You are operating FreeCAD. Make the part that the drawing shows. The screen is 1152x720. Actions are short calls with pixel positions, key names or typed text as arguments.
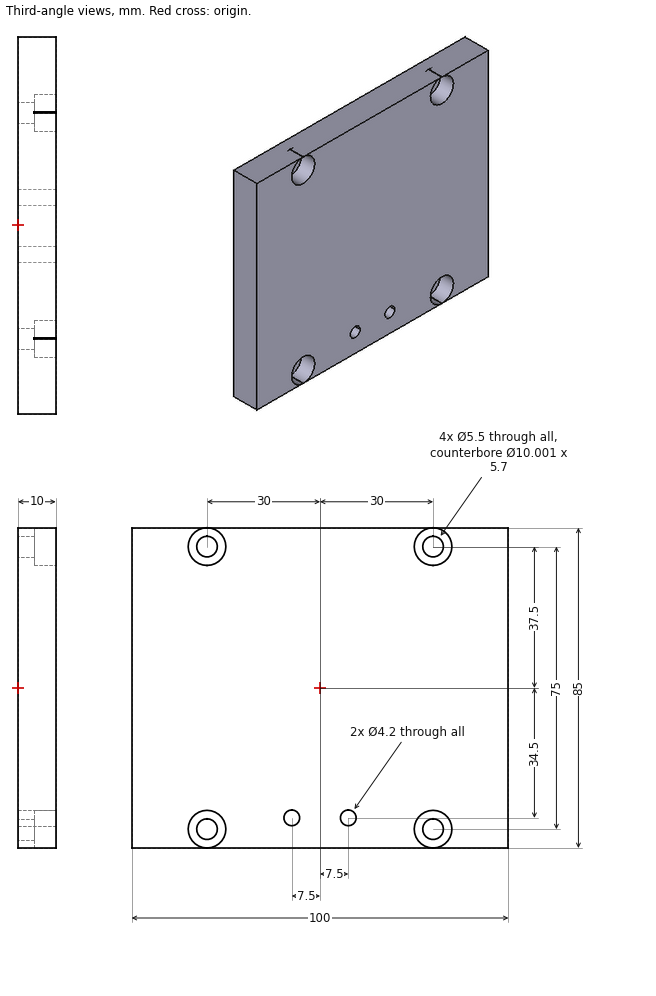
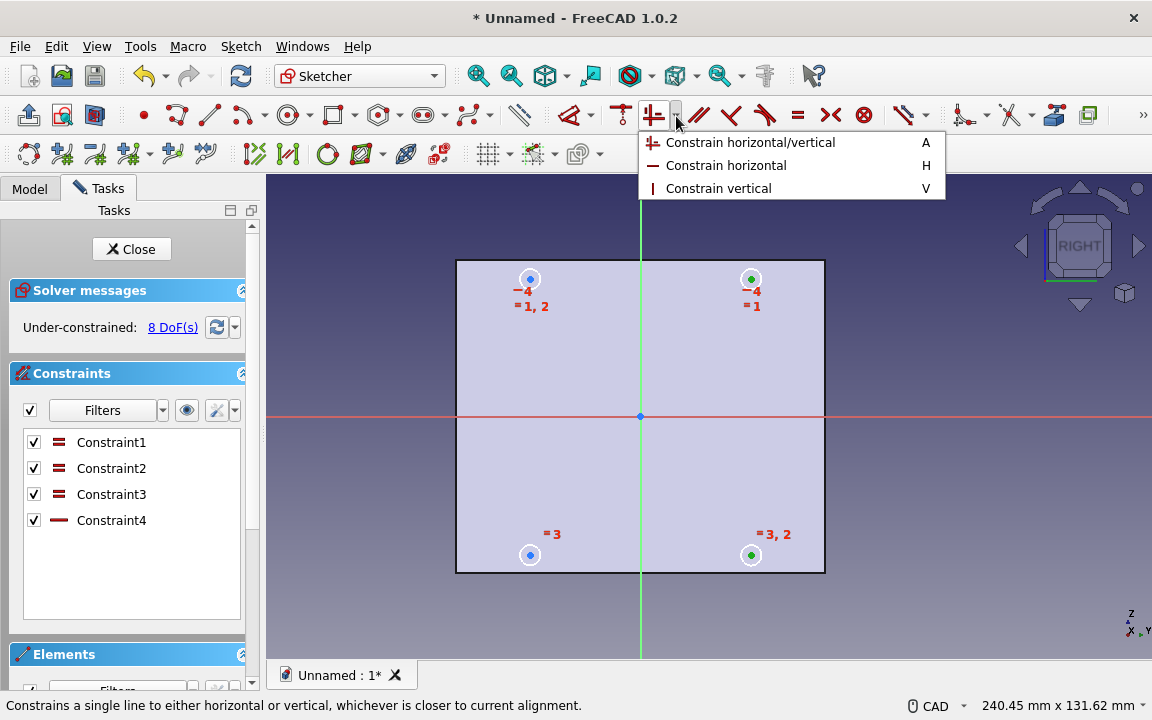
click(792, 188)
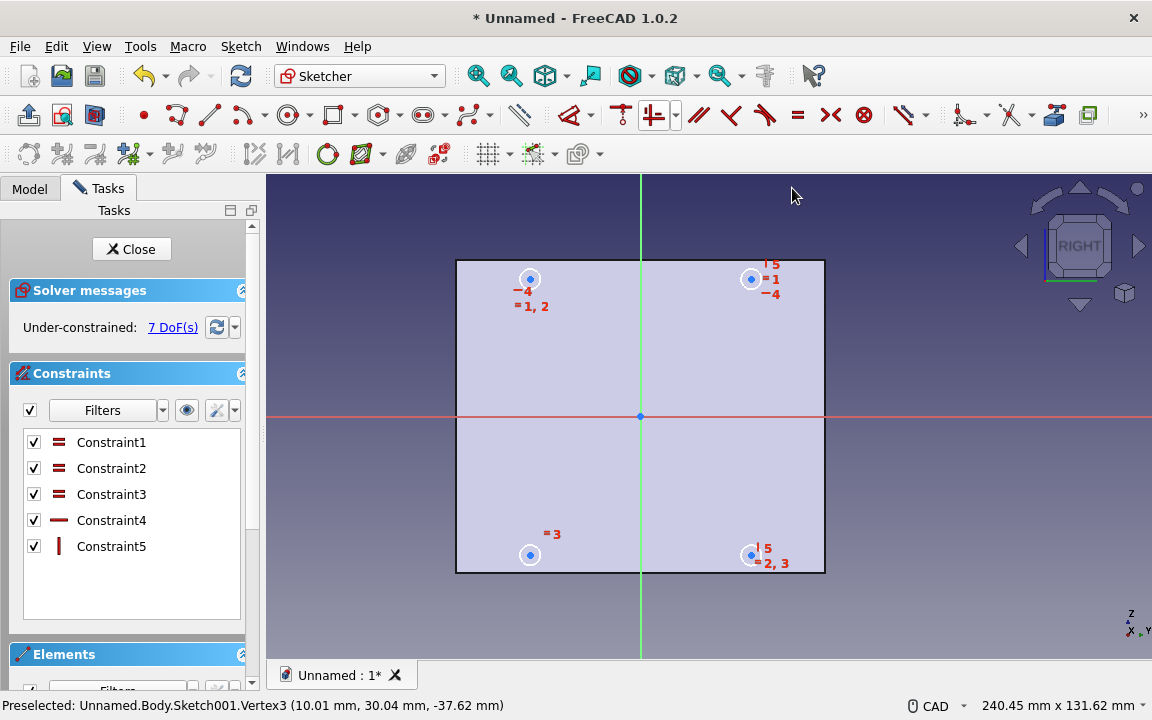
click(530, 279)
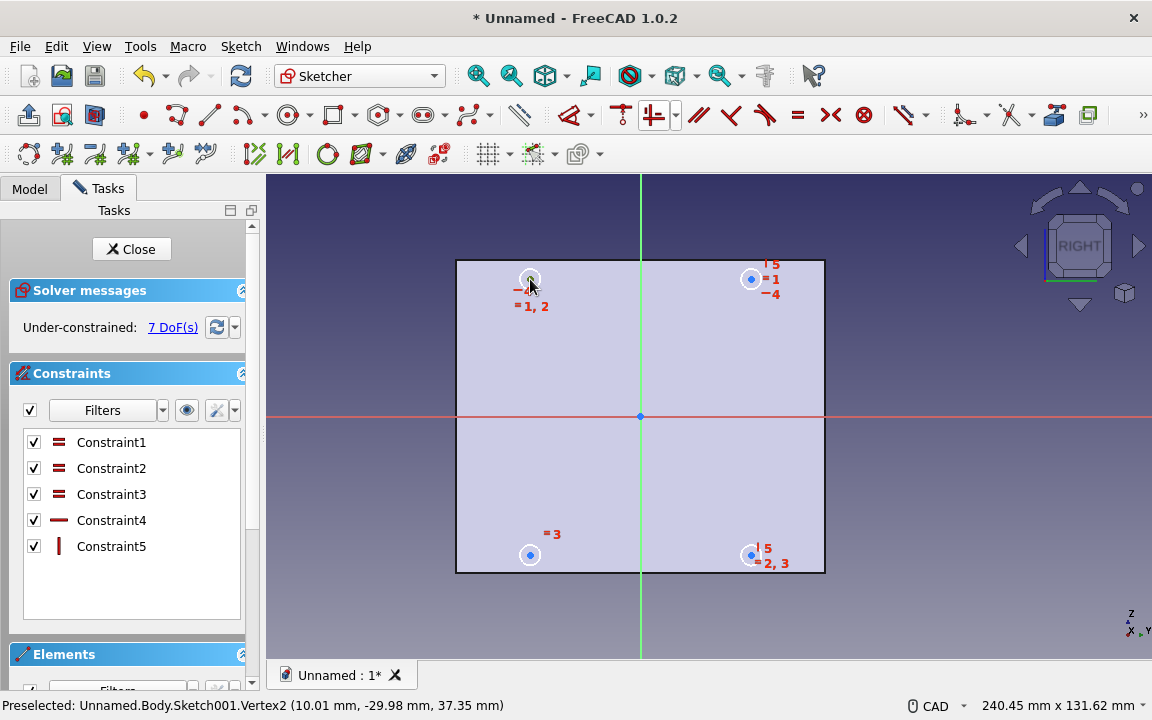
click(530, 555)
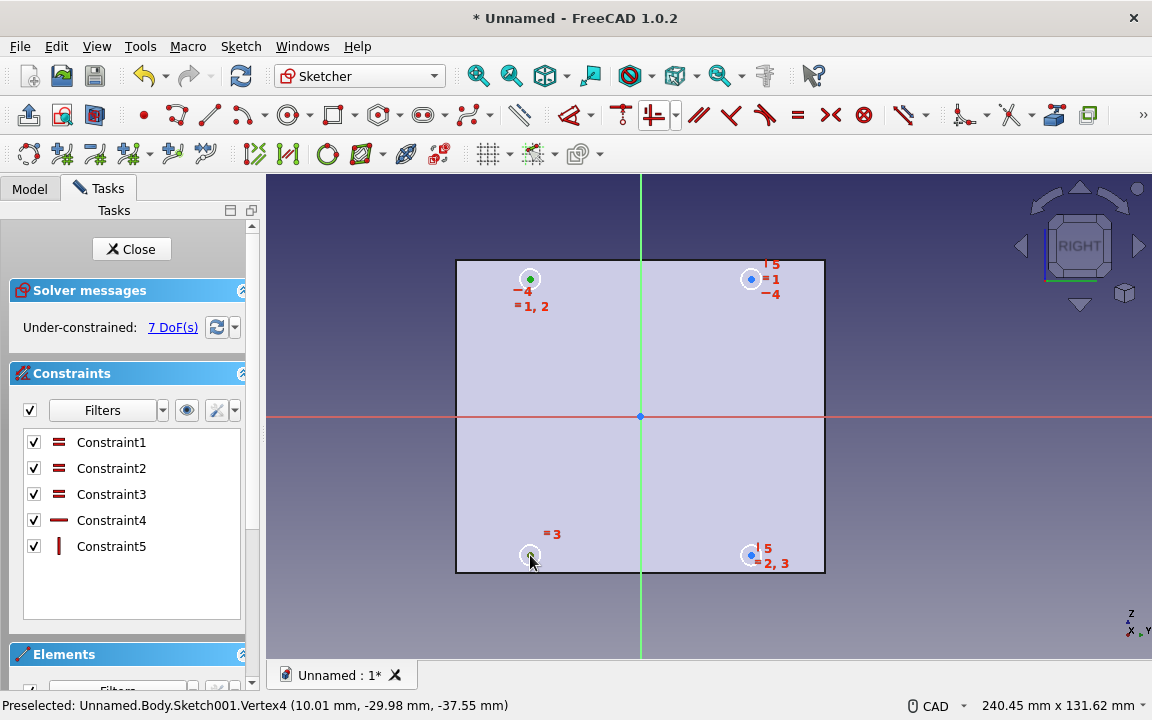
click(676, 116)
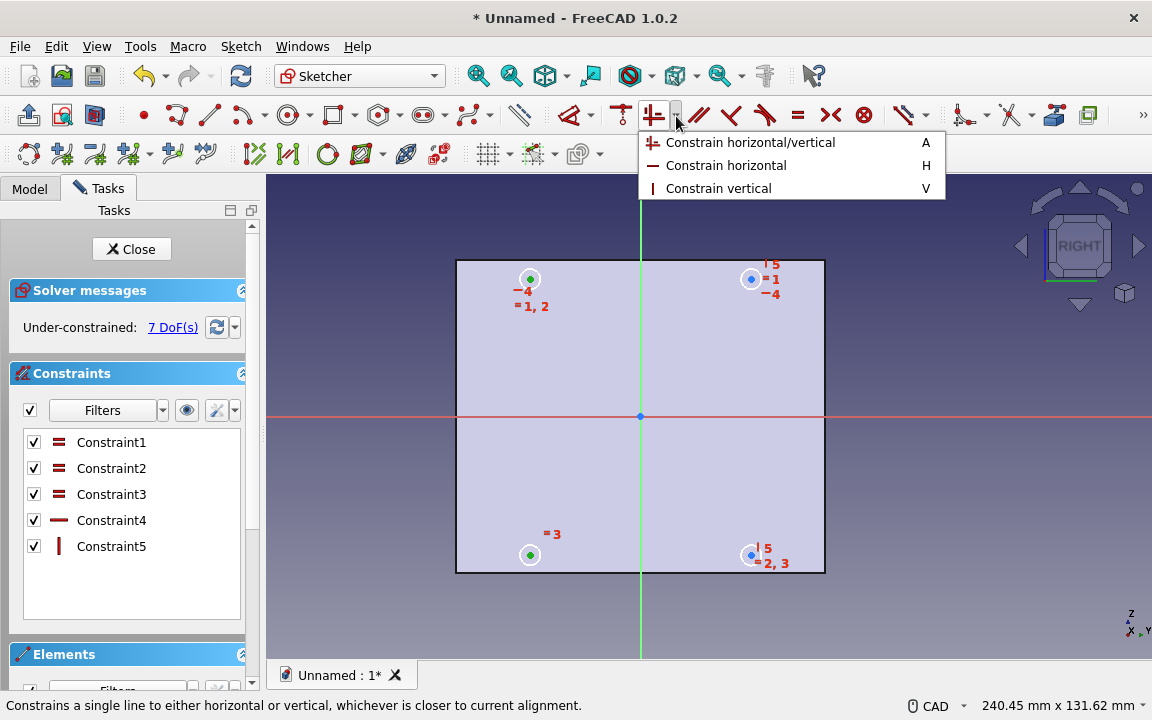
click(792, 188)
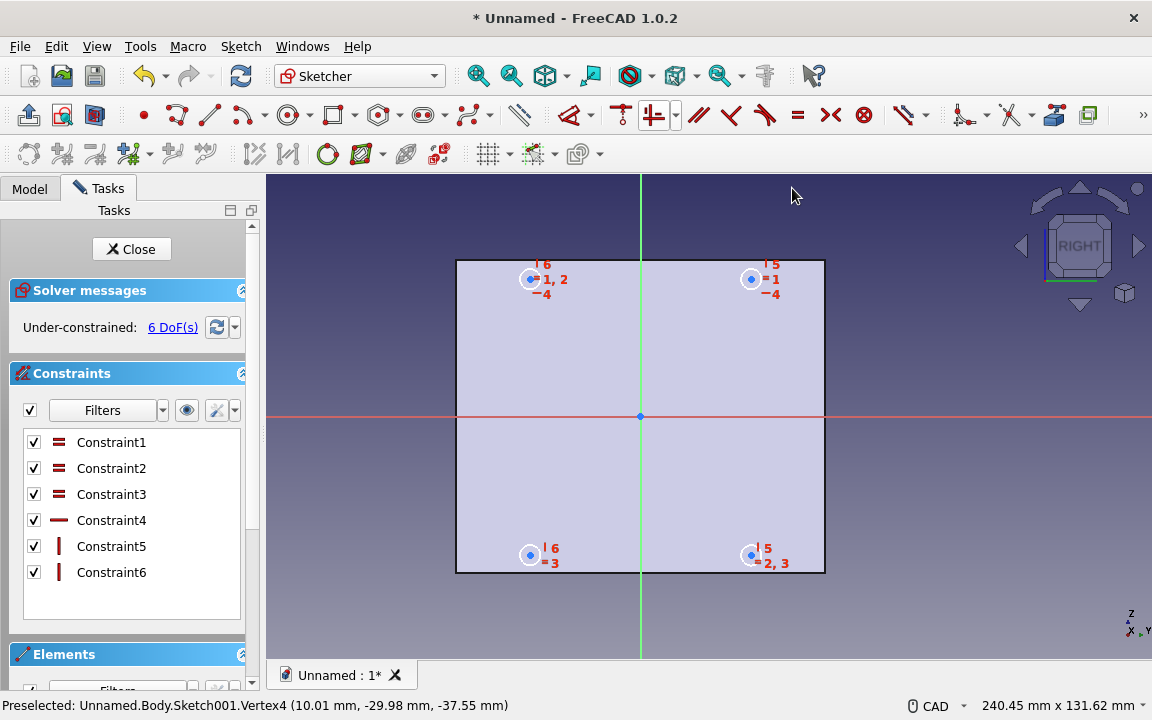
click(751, 555)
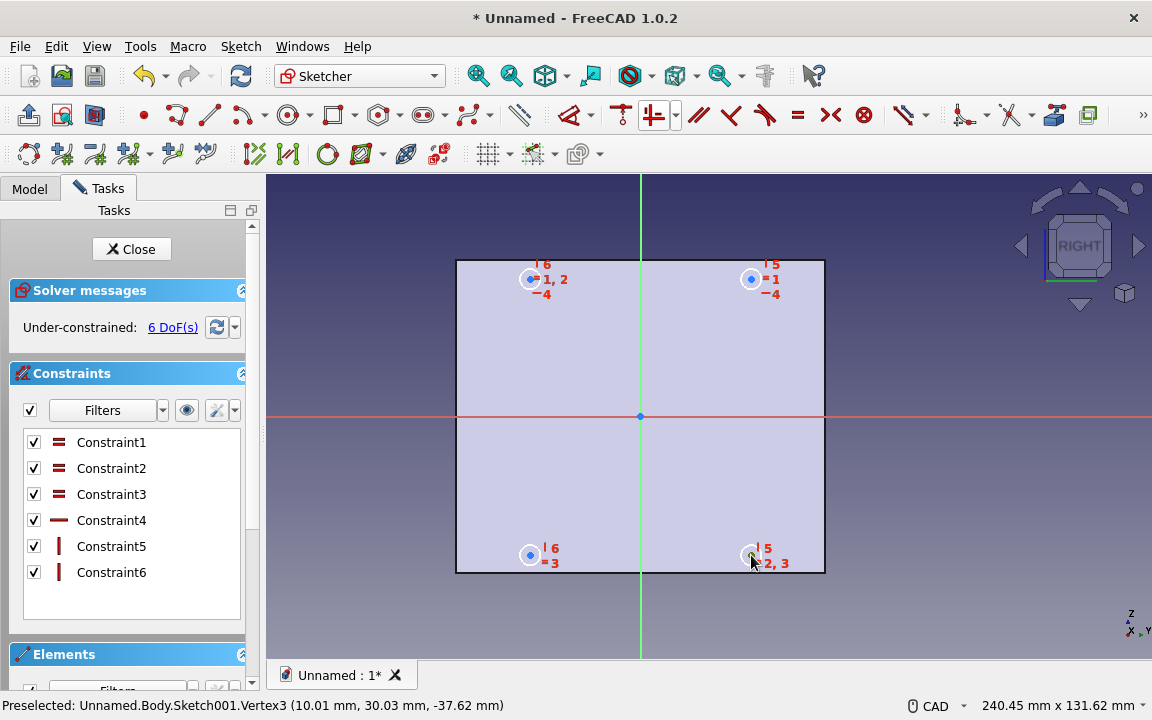
click(530, 555)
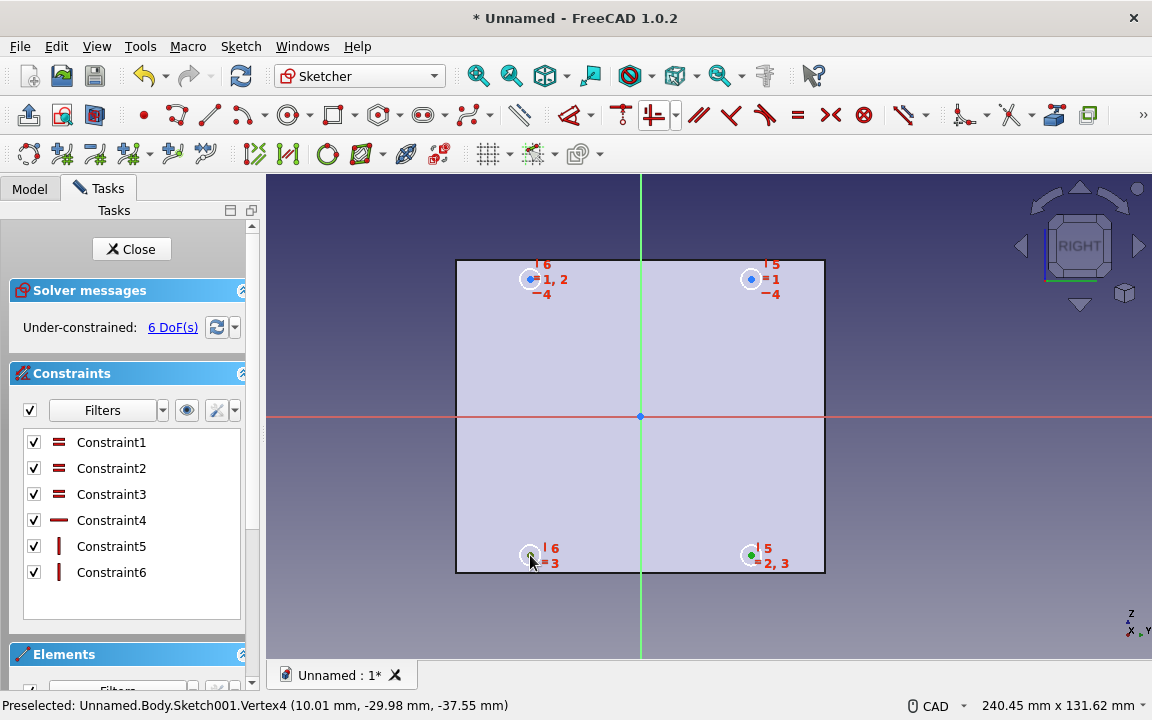
click(676, 116)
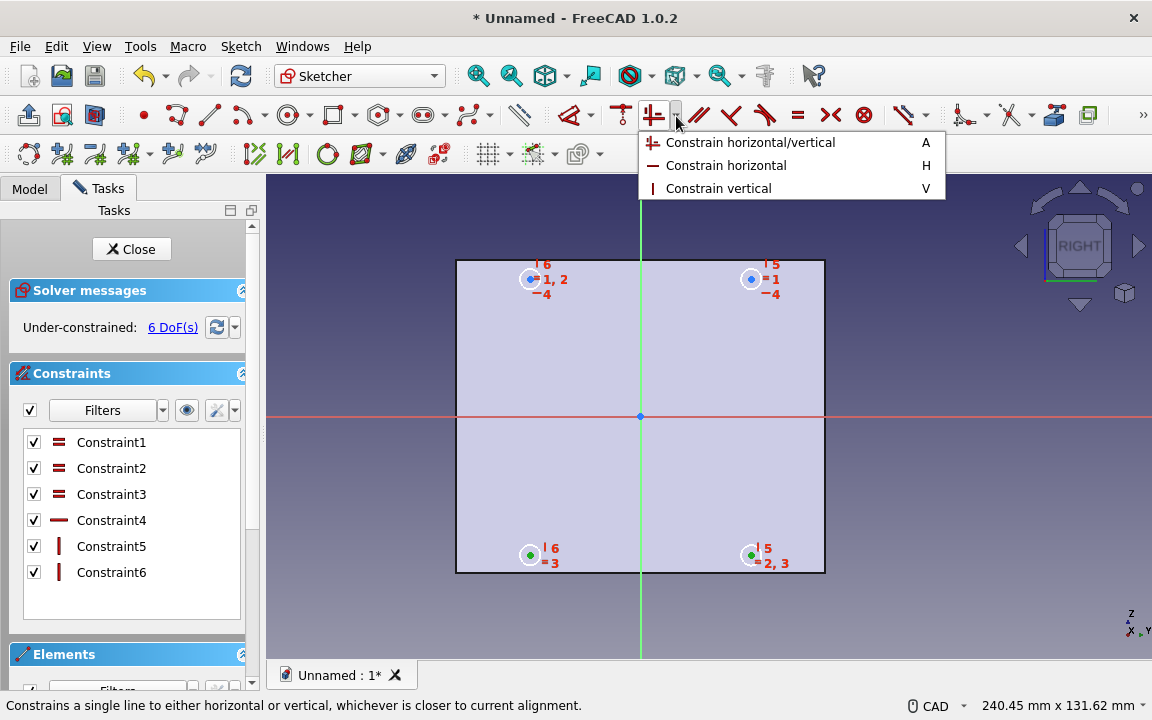
click(792, 166)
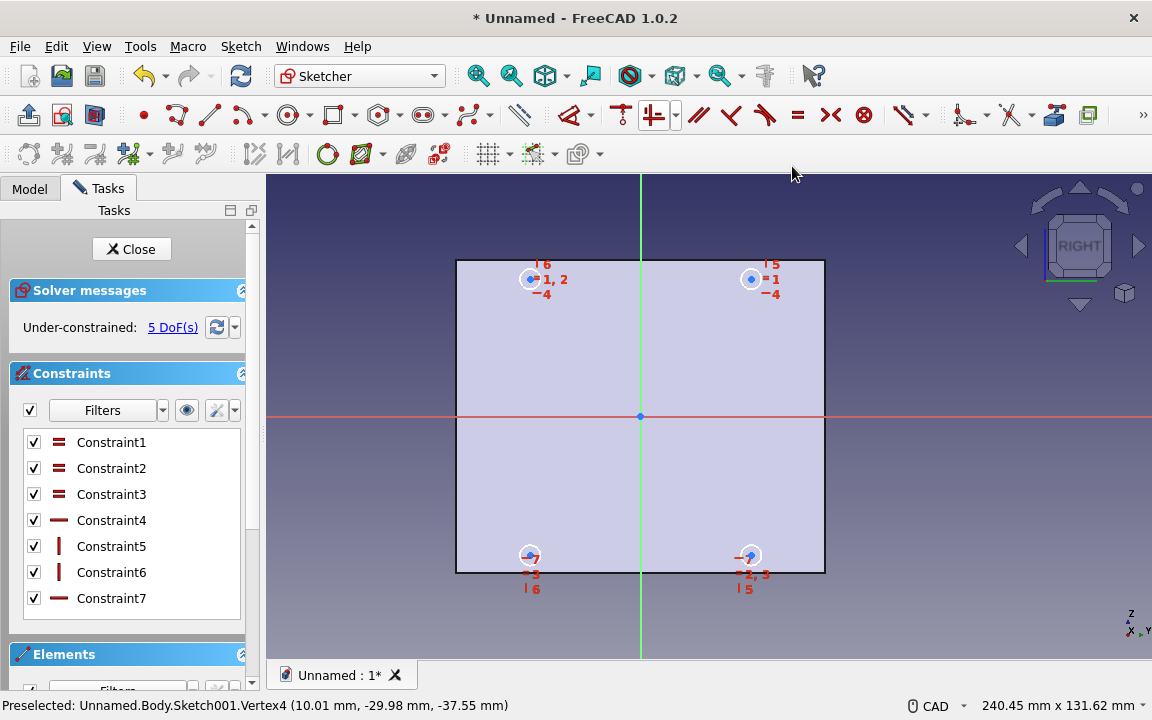
click(568, 116)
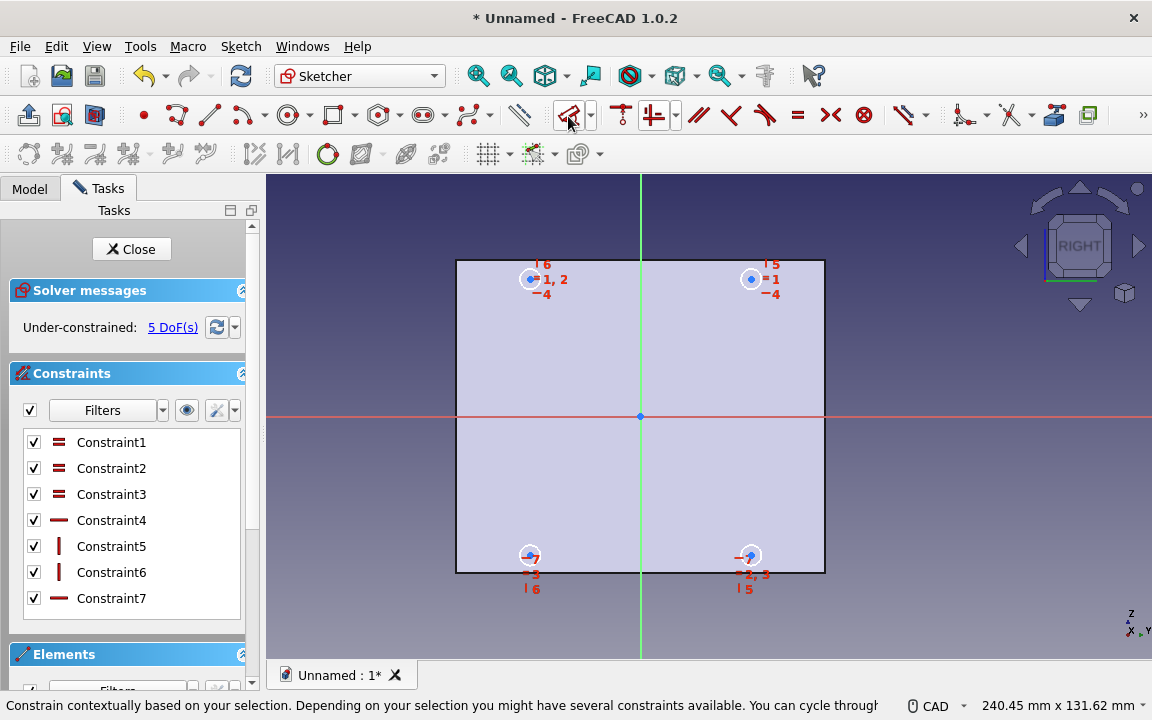
scroll(758, 272, up, 4)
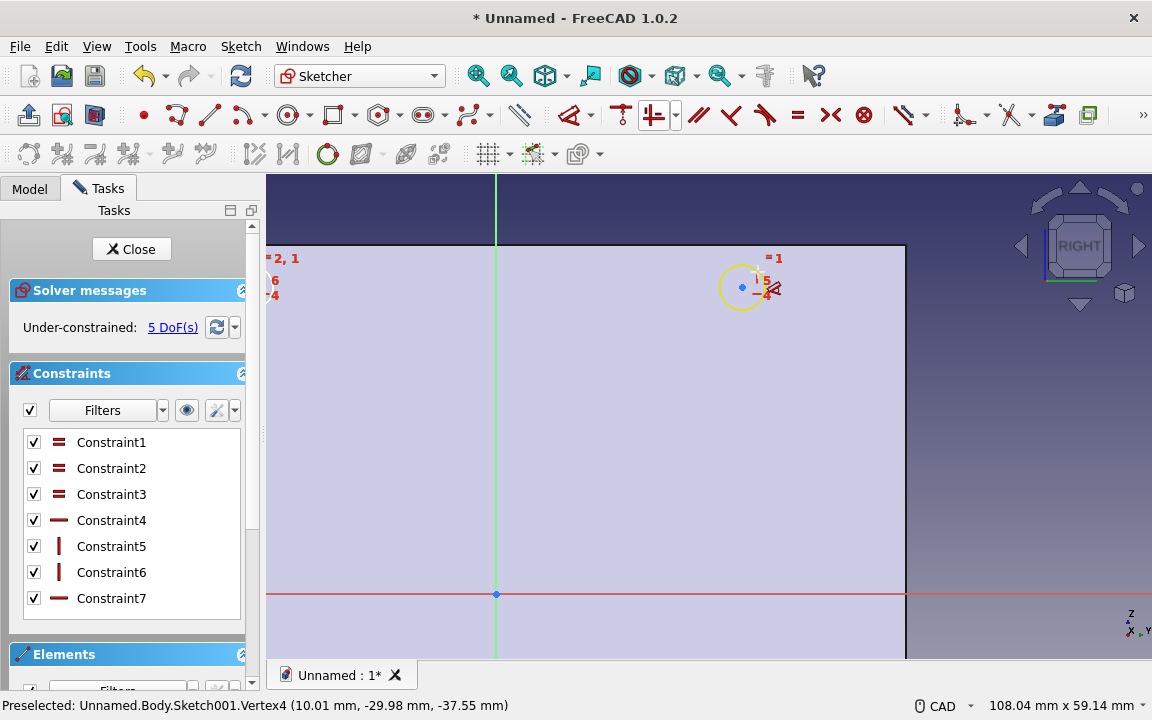
click(758, 272)
click(781, 249)